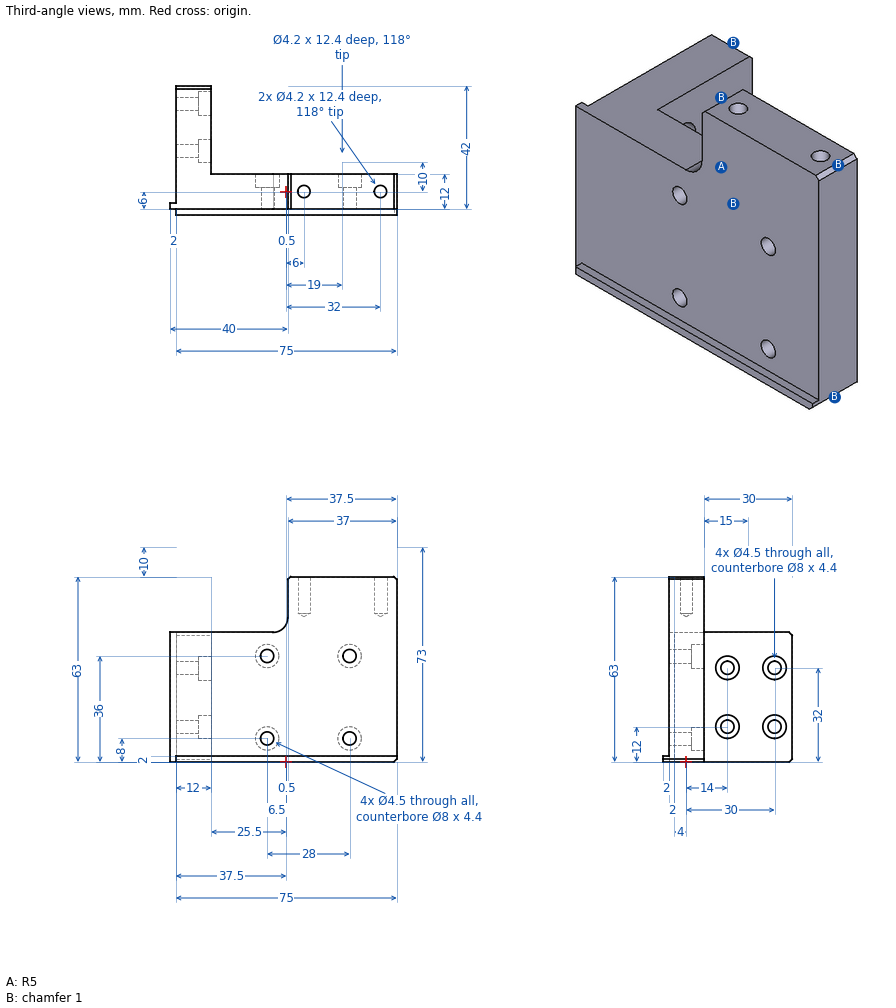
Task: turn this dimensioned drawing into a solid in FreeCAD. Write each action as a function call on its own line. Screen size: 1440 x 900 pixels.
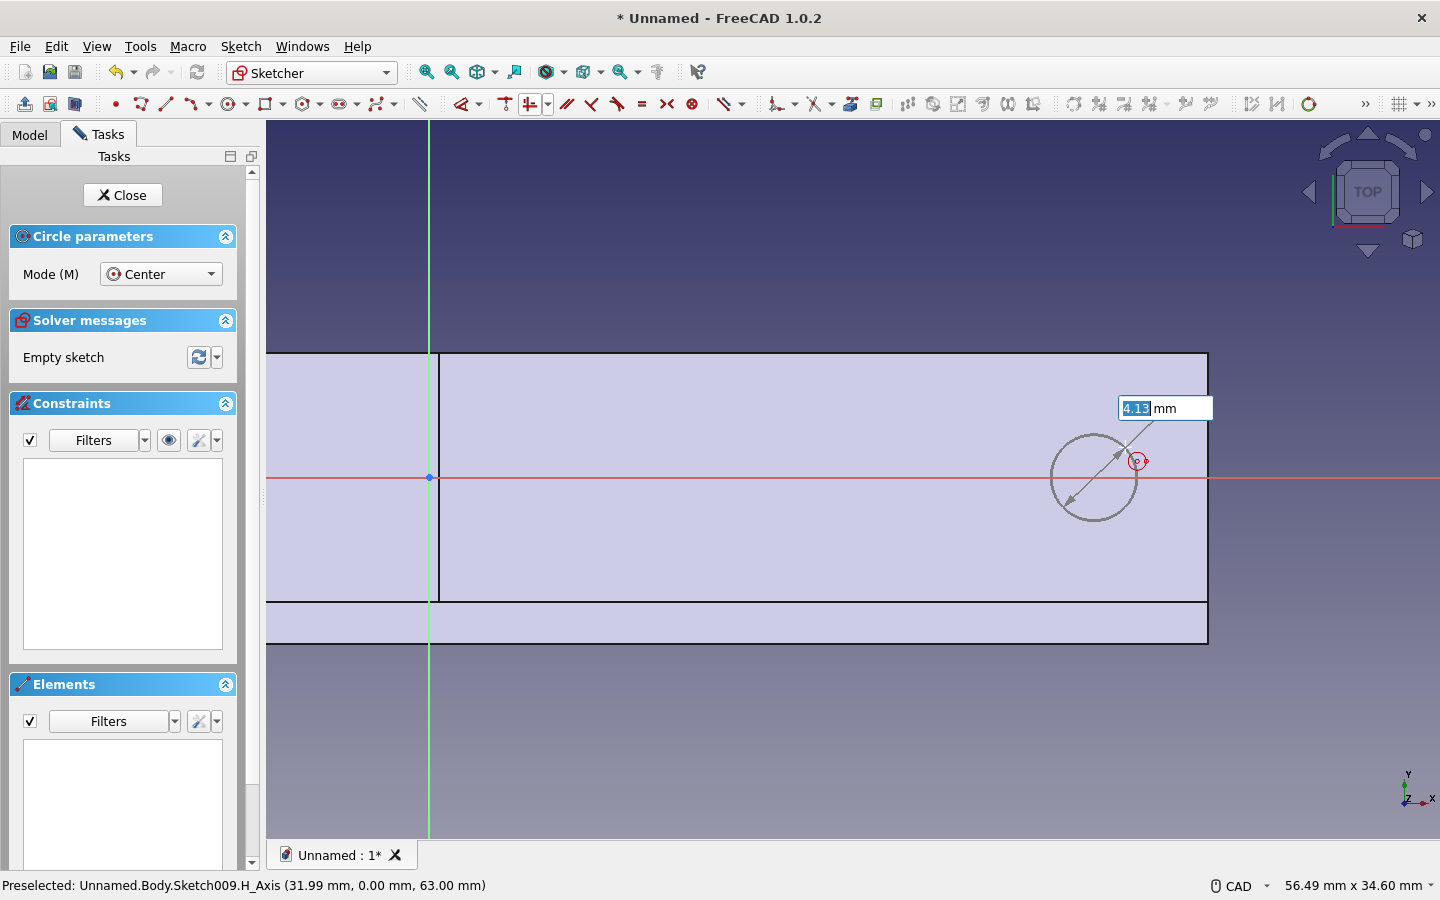
text(4.2)
key(Return)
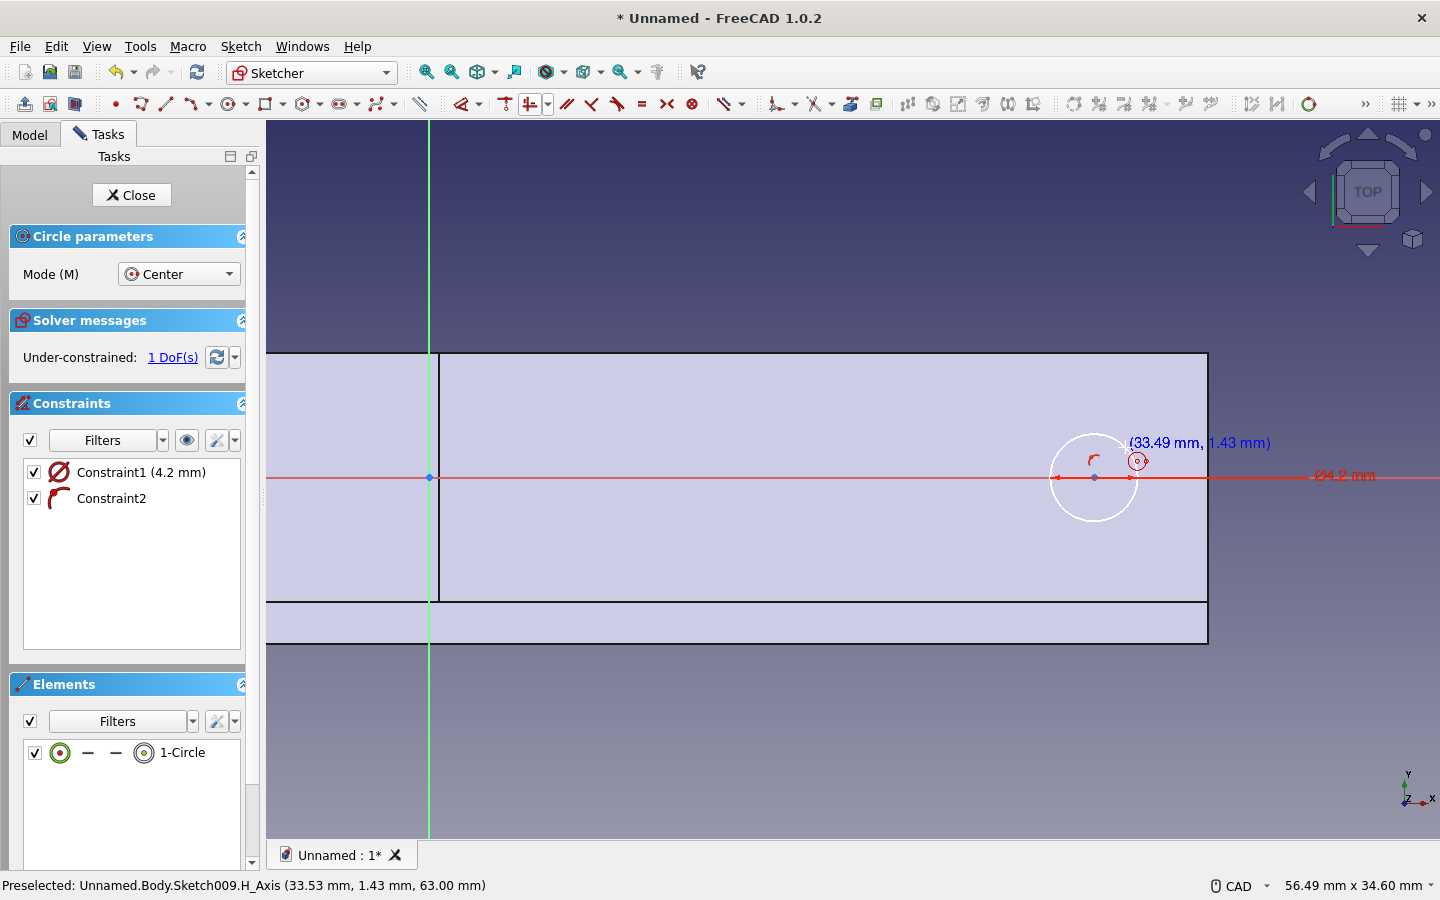
click(554, 478)
move(585, 447)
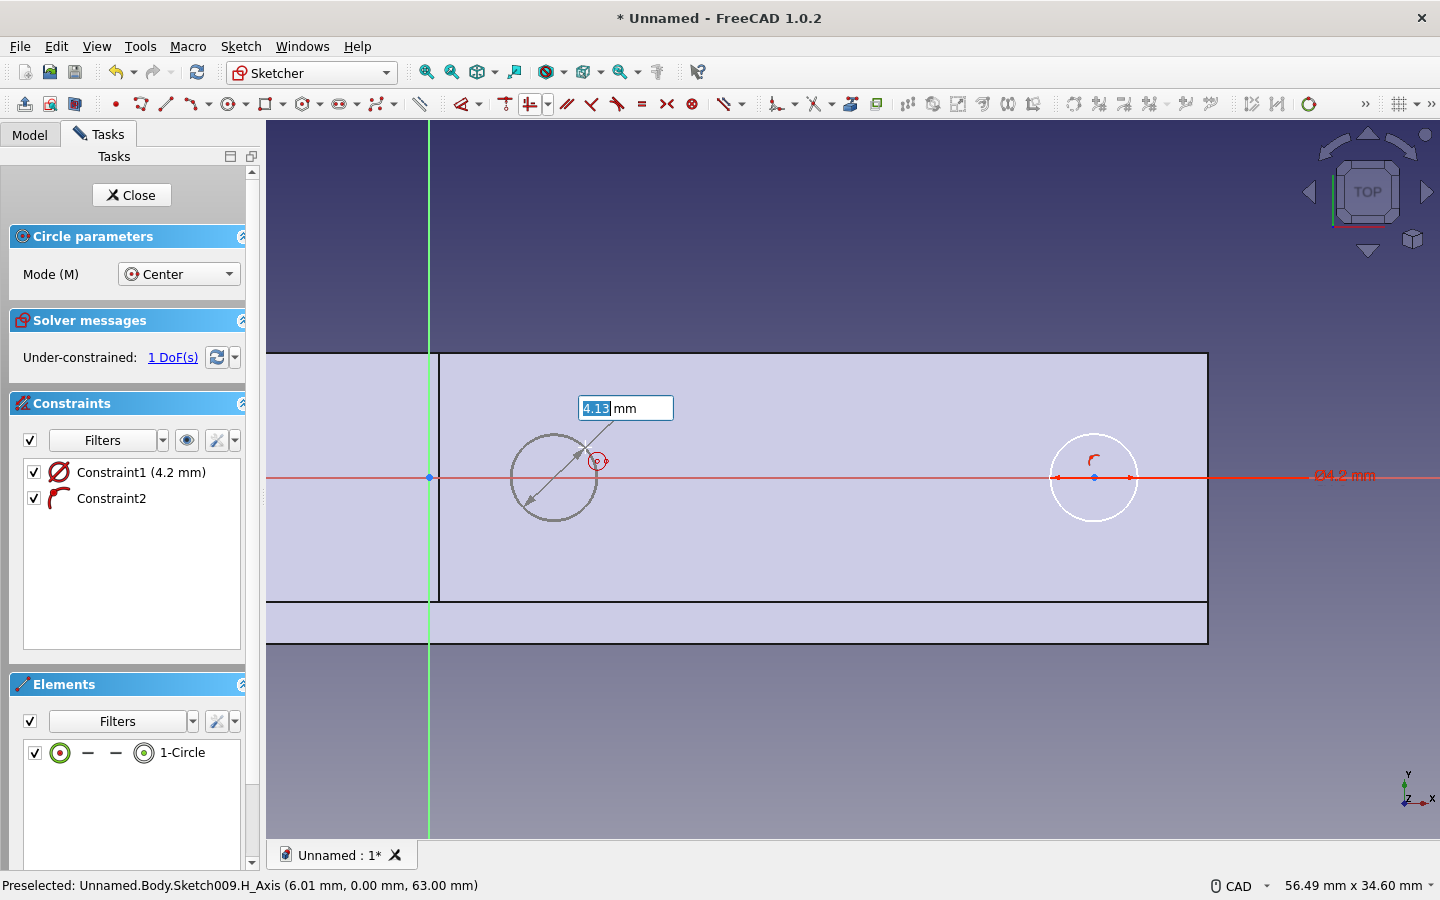
text(4.2)
key(Return)
key(Escape)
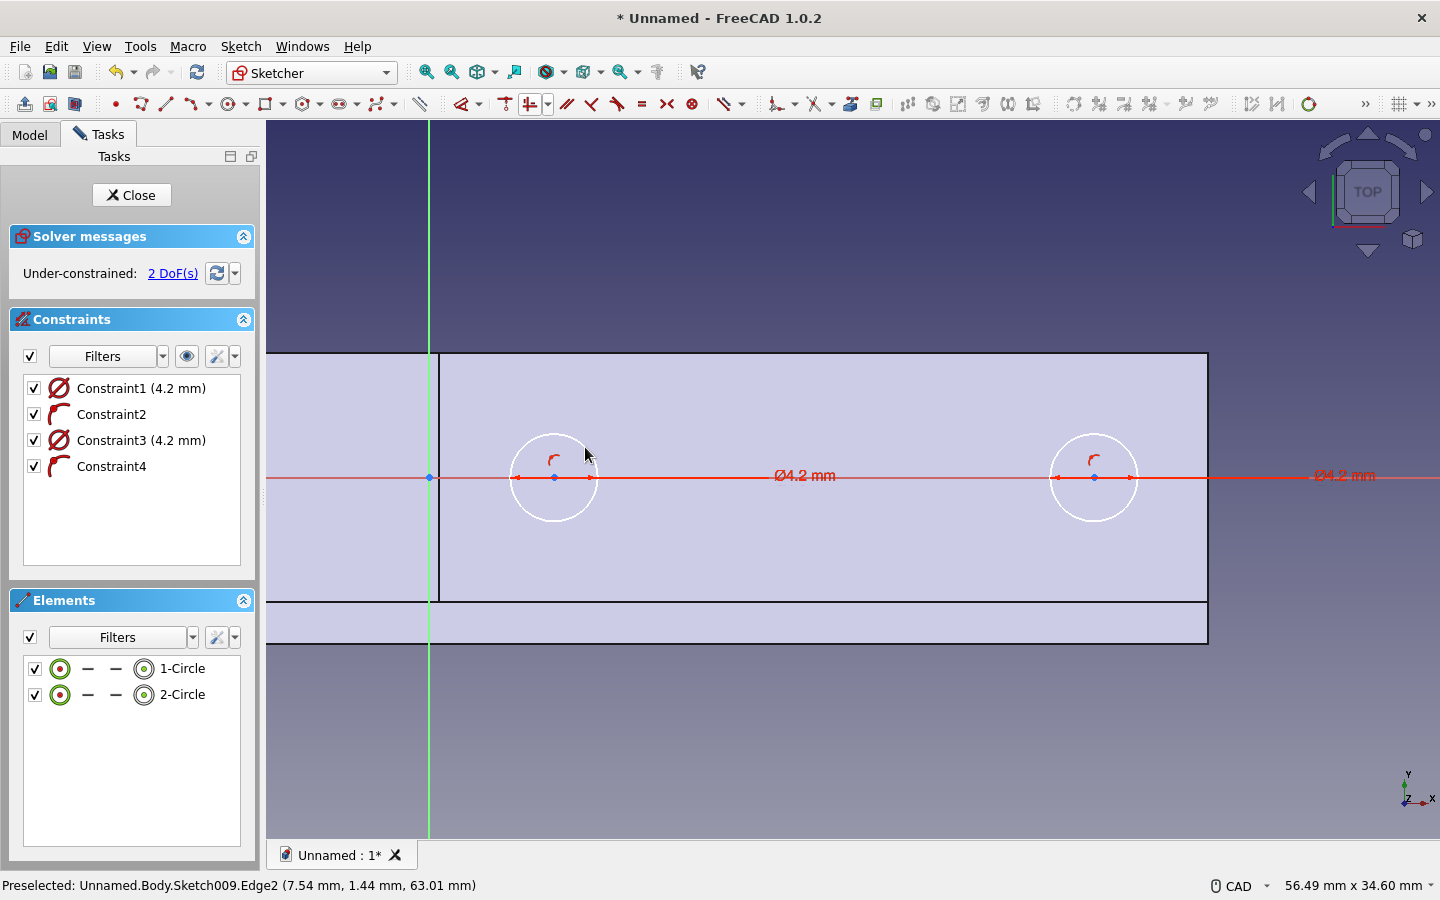
click(460, 104)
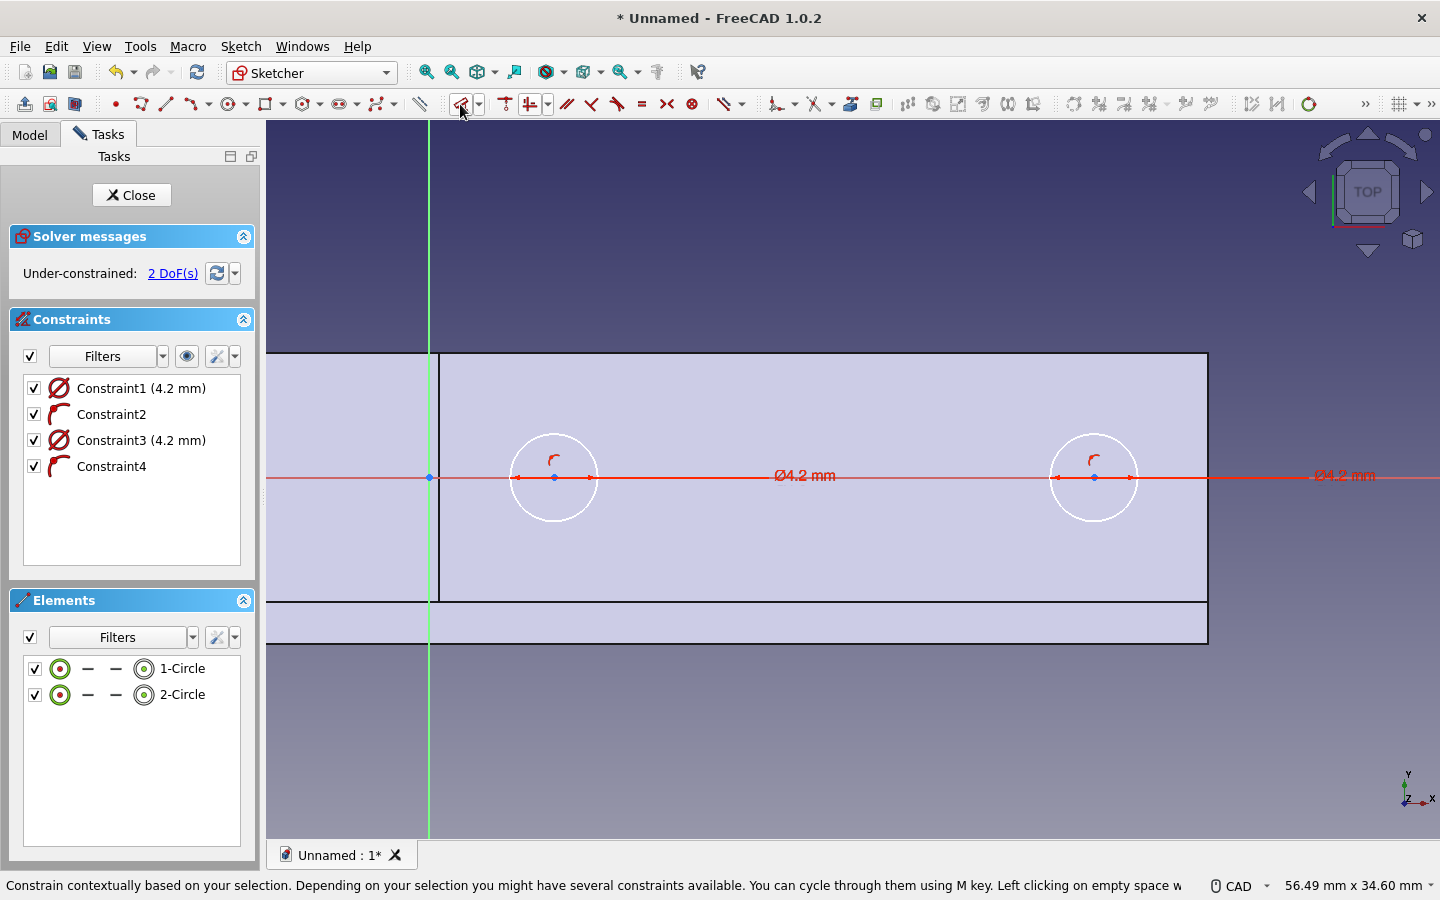
click(554, 478)
click(492, 512)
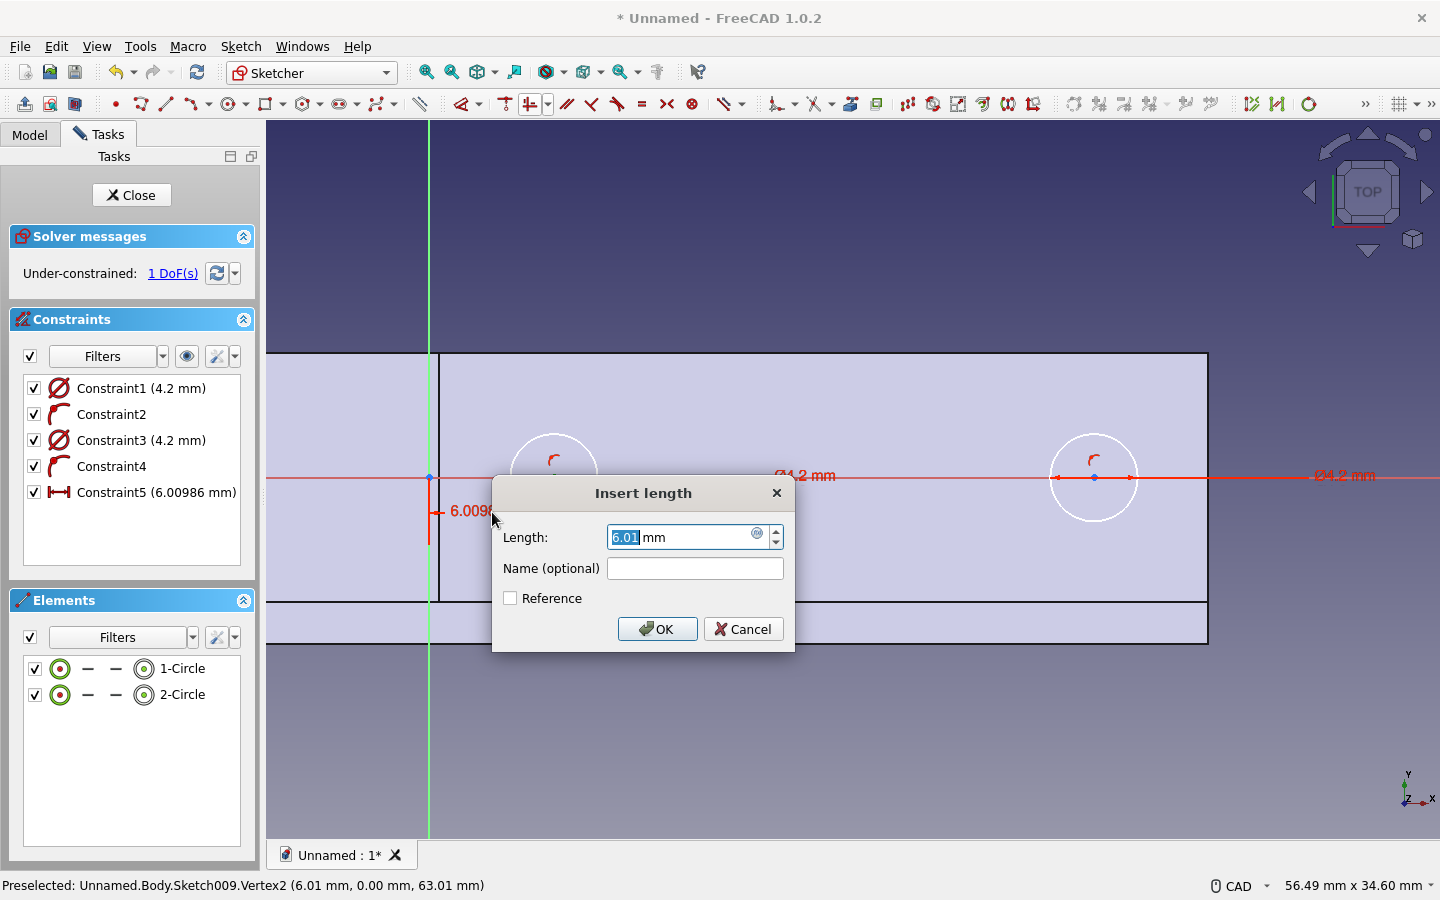
text(6)
key(Return)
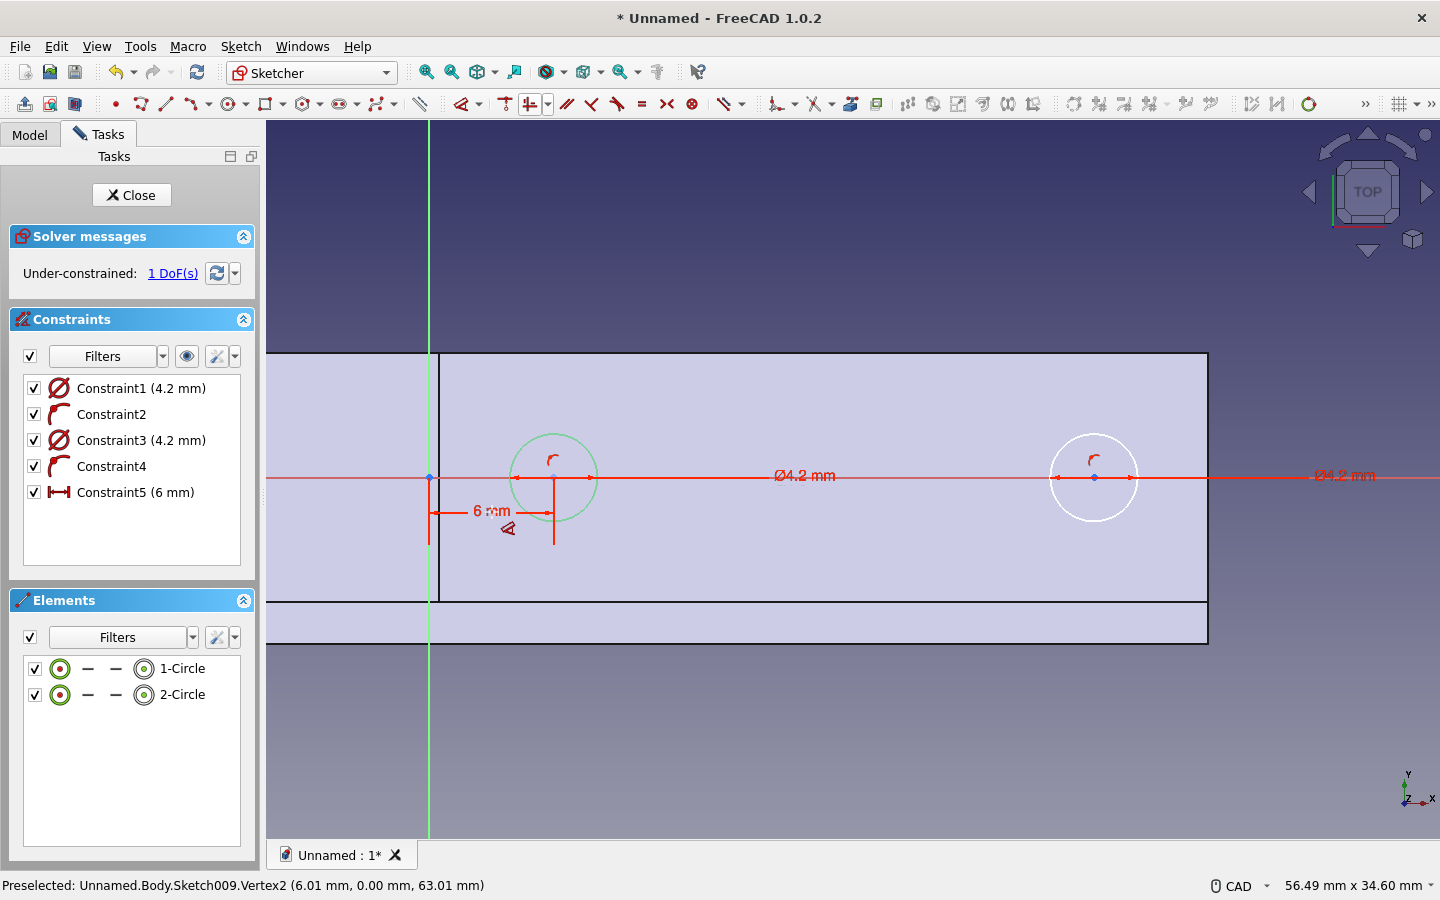
click(1094, 478)
click(762, 512)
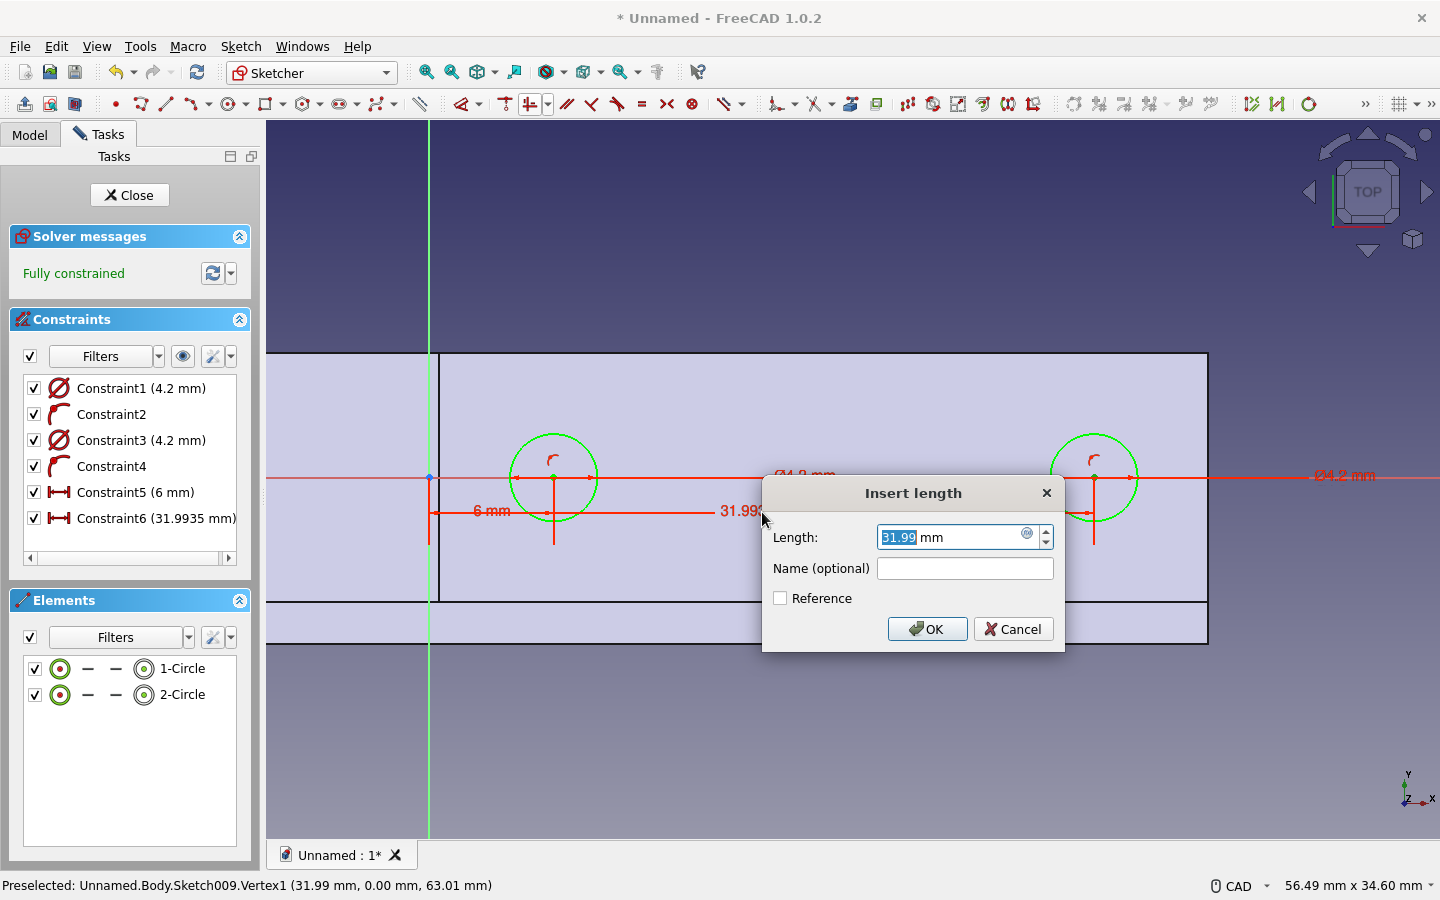
text(32)
key(Return)
key(Escape)